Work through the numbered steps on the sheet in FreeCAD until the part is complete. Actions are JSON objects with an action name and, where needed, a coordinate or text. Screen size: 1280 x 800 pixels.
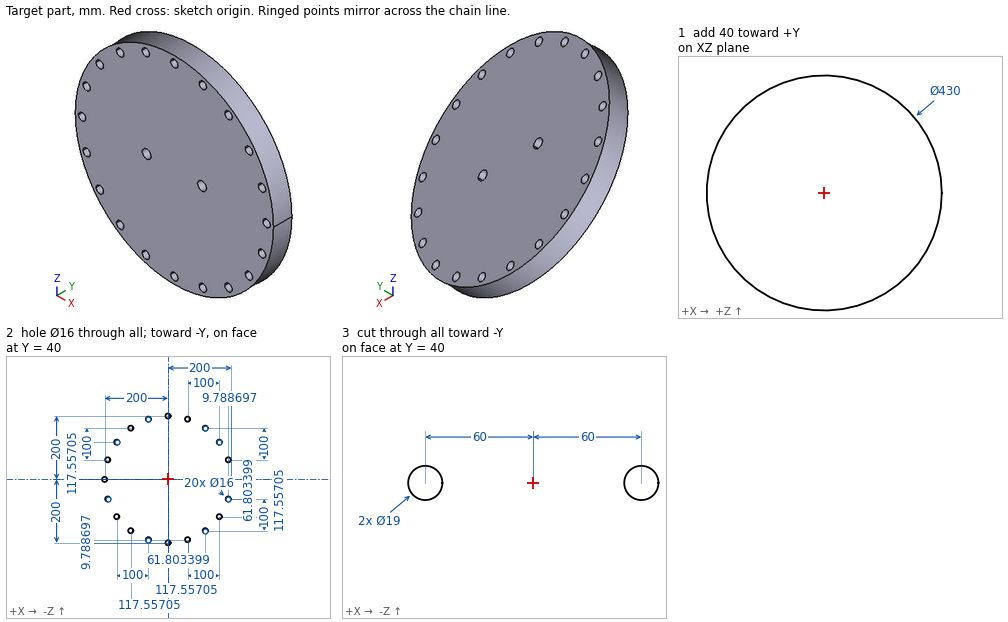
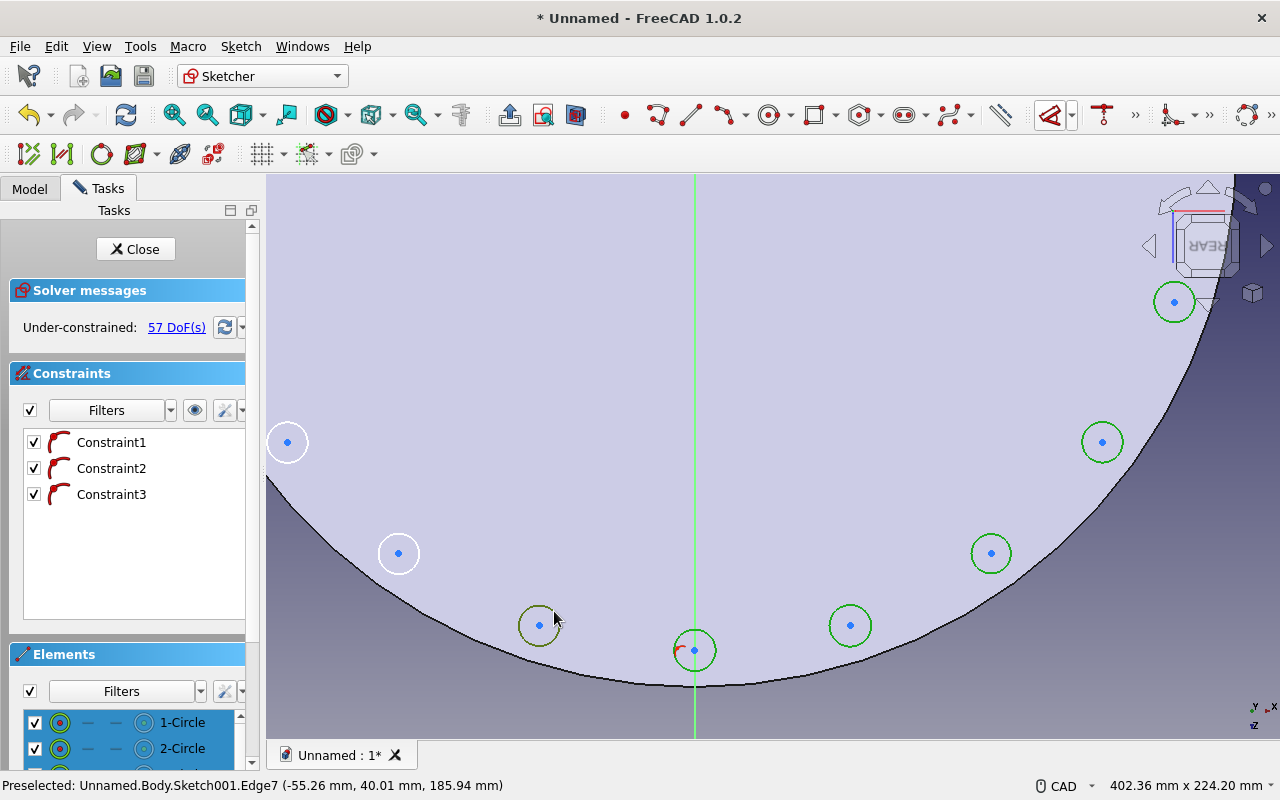
{"action": "left_click", "coordinate": [413, 540]}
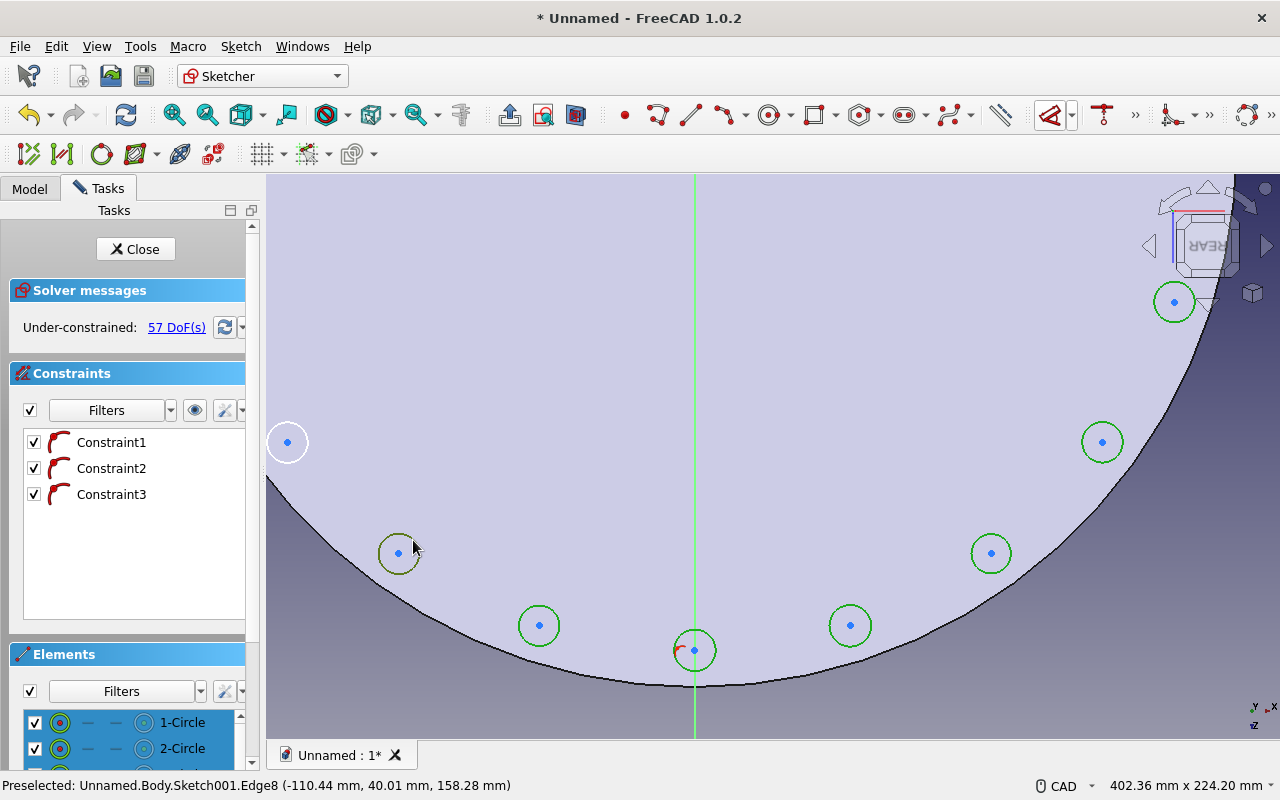
{"action": "left_click", "coordinate": [302, 428]}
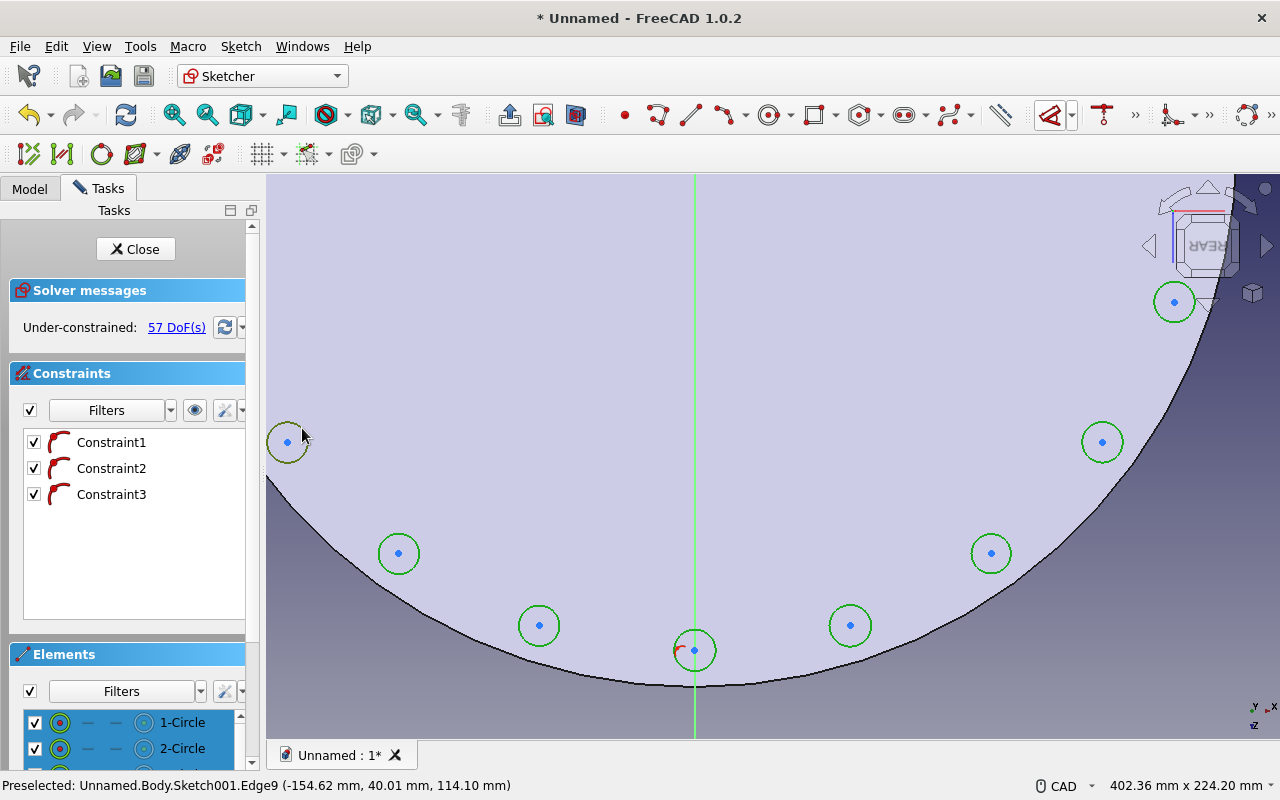
{"action": "scroll", "coordinate": [710, 638], "scroll_direction": "down", "scroll_amount": 5}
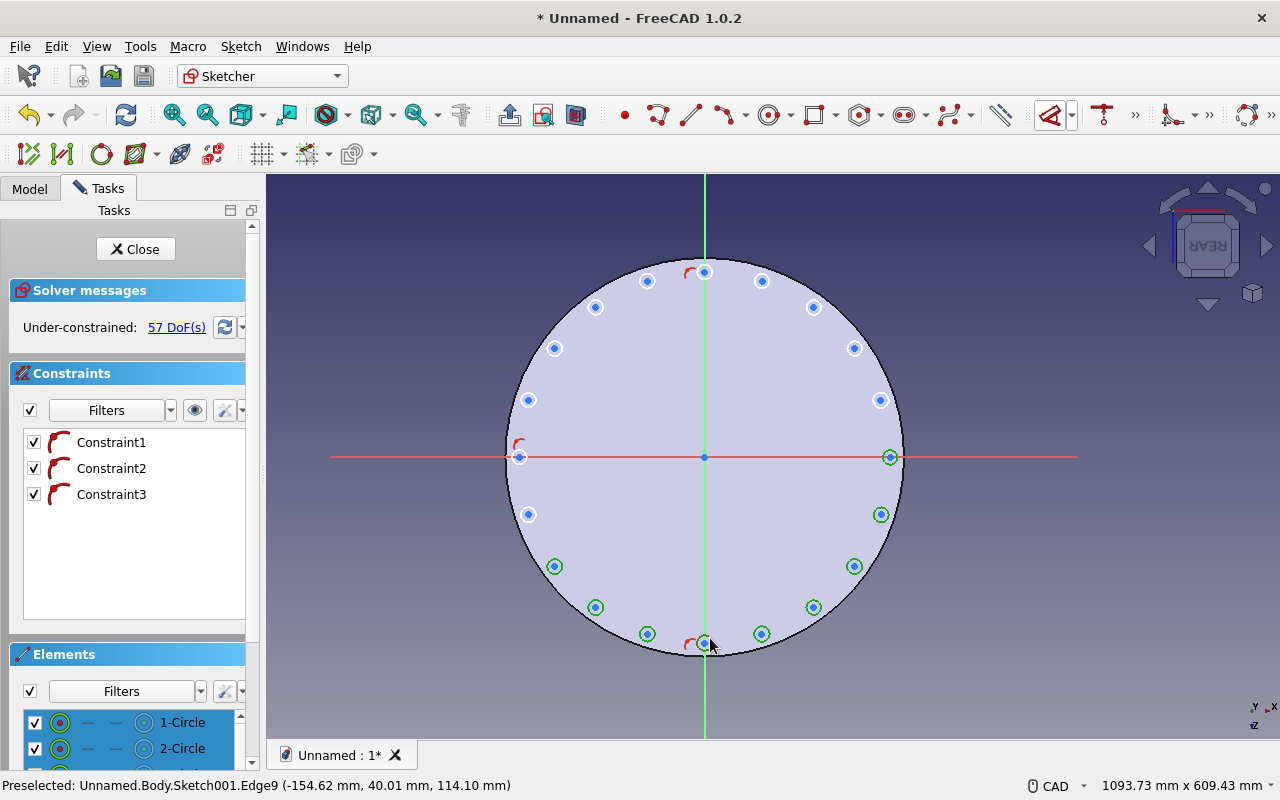
{"action": "scroll", "coordinate": [534, 510], "scroll_direction": "up", "scroll_amount": 4}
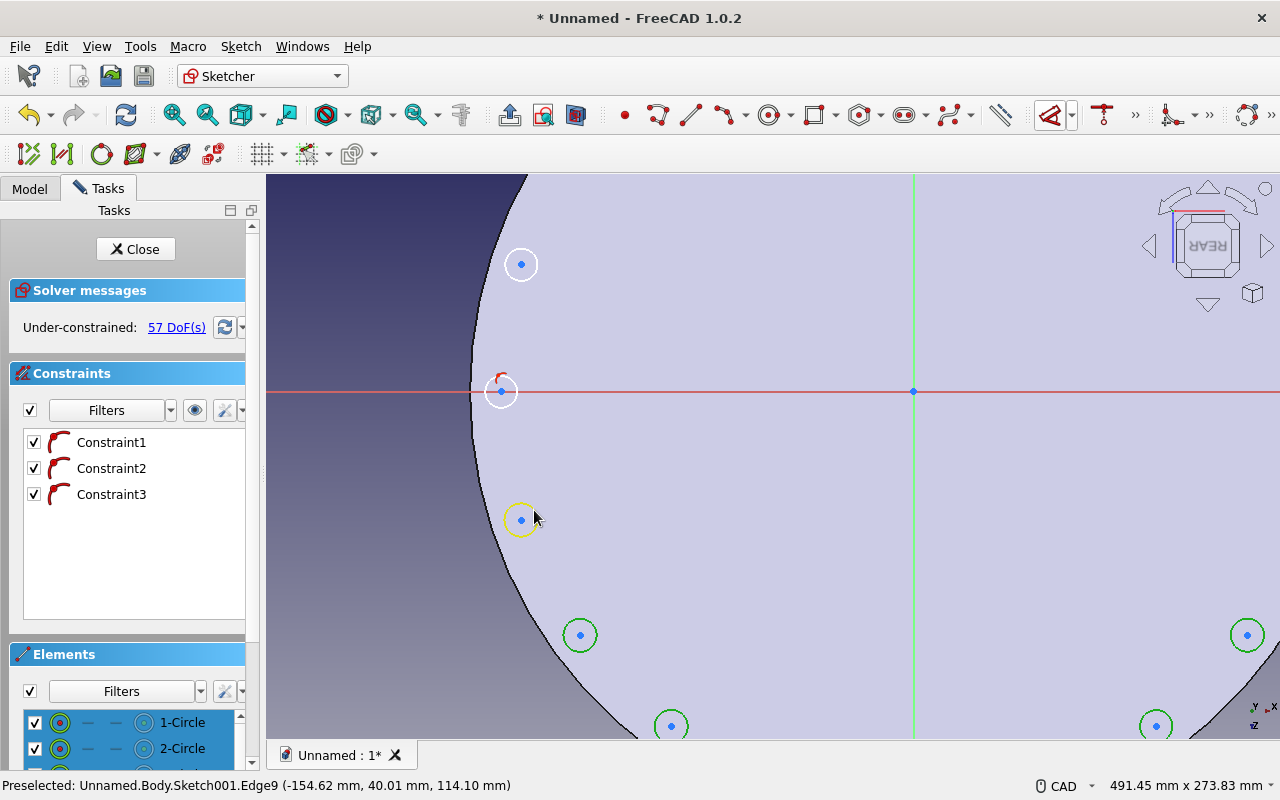
{"action": "left_click", "coordinate": [533, 508]}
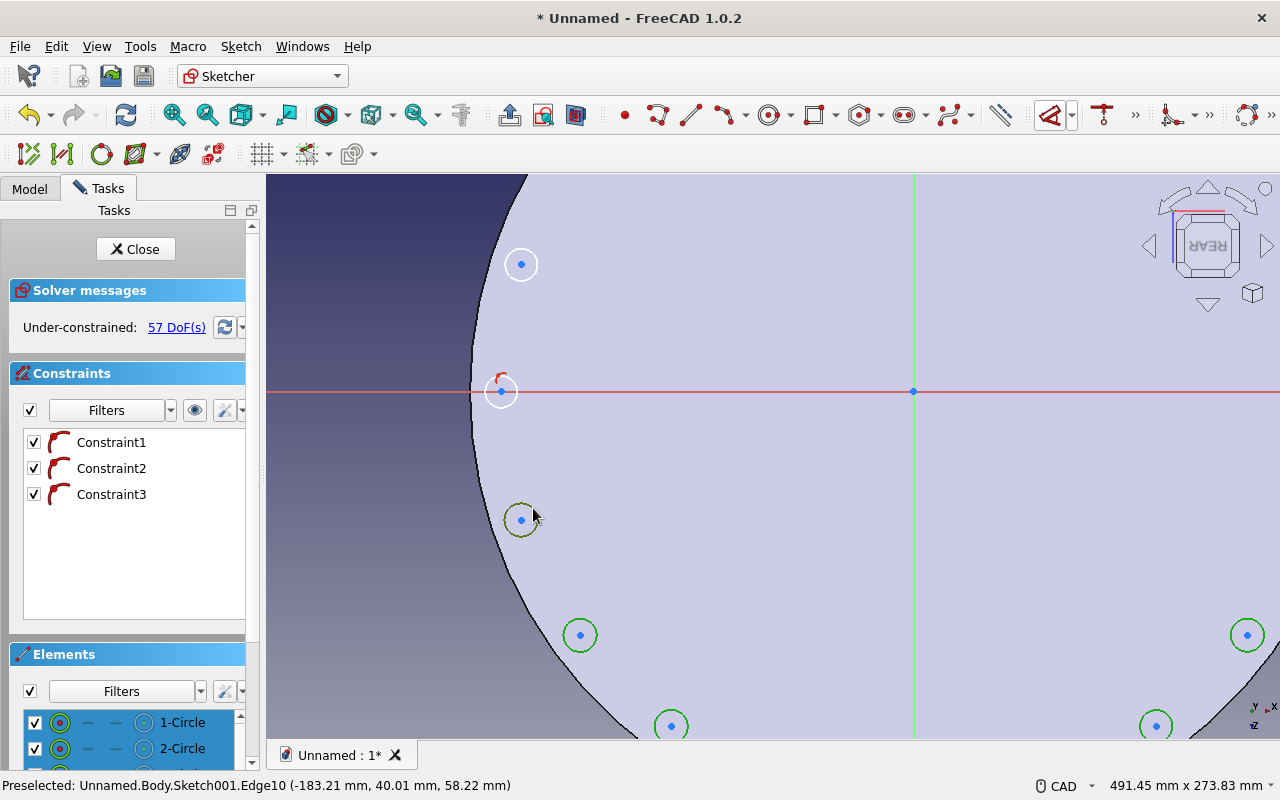
{"action": "scroll", "coordinate": [512, 381], "scroll_direction": "up", "scroll_amount": 2}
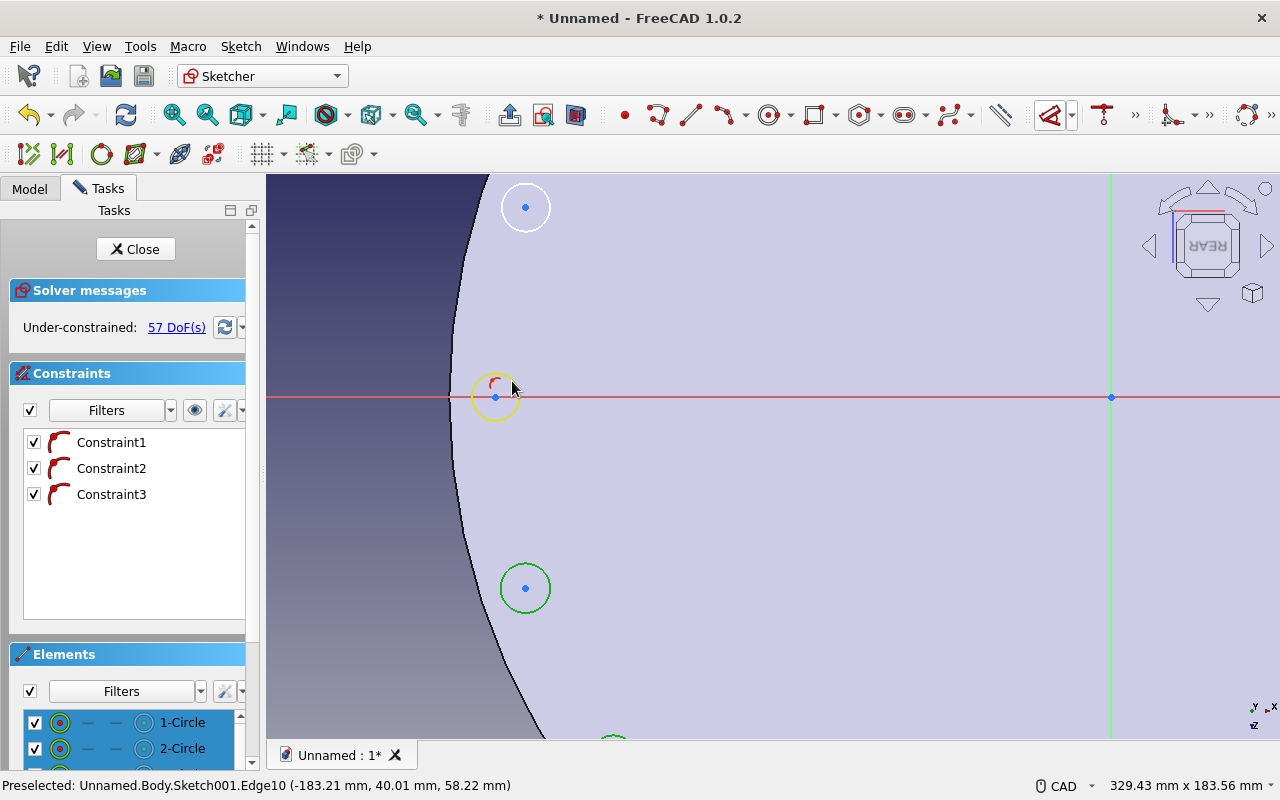
{"action": "left_click", "coordinate": [513, 380]}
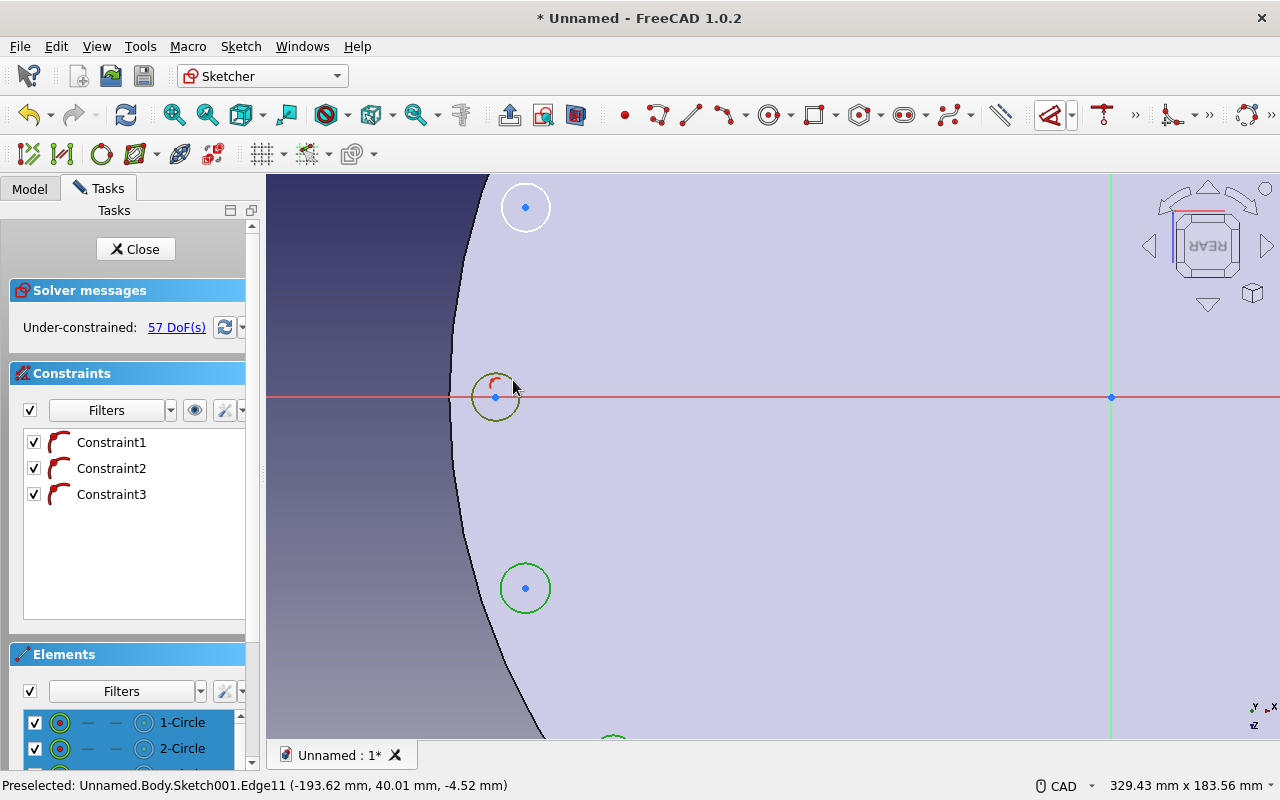
{"action": "left_click", "coordinate": [509, 225]}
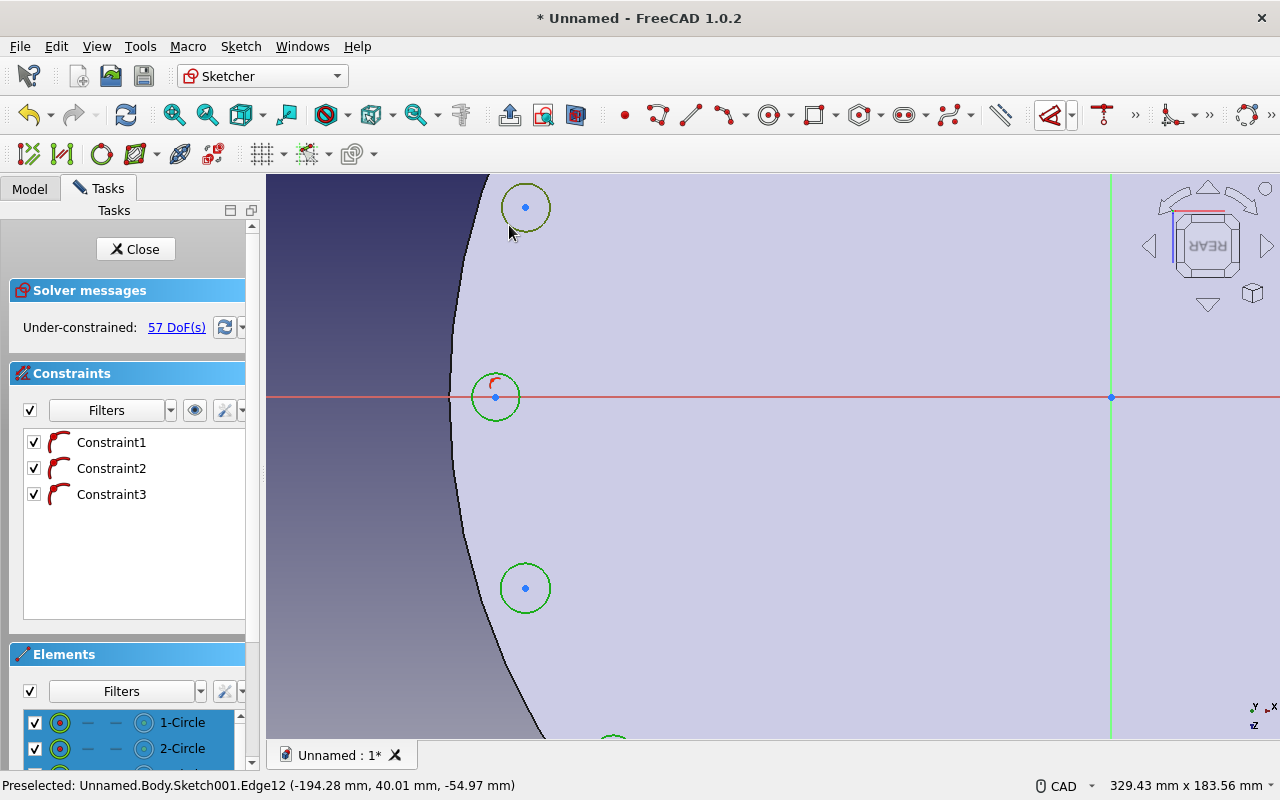
{"action": "scroll", "coordinate": [529, 482], "scroll_direction": "down", "scroll_amount": 6}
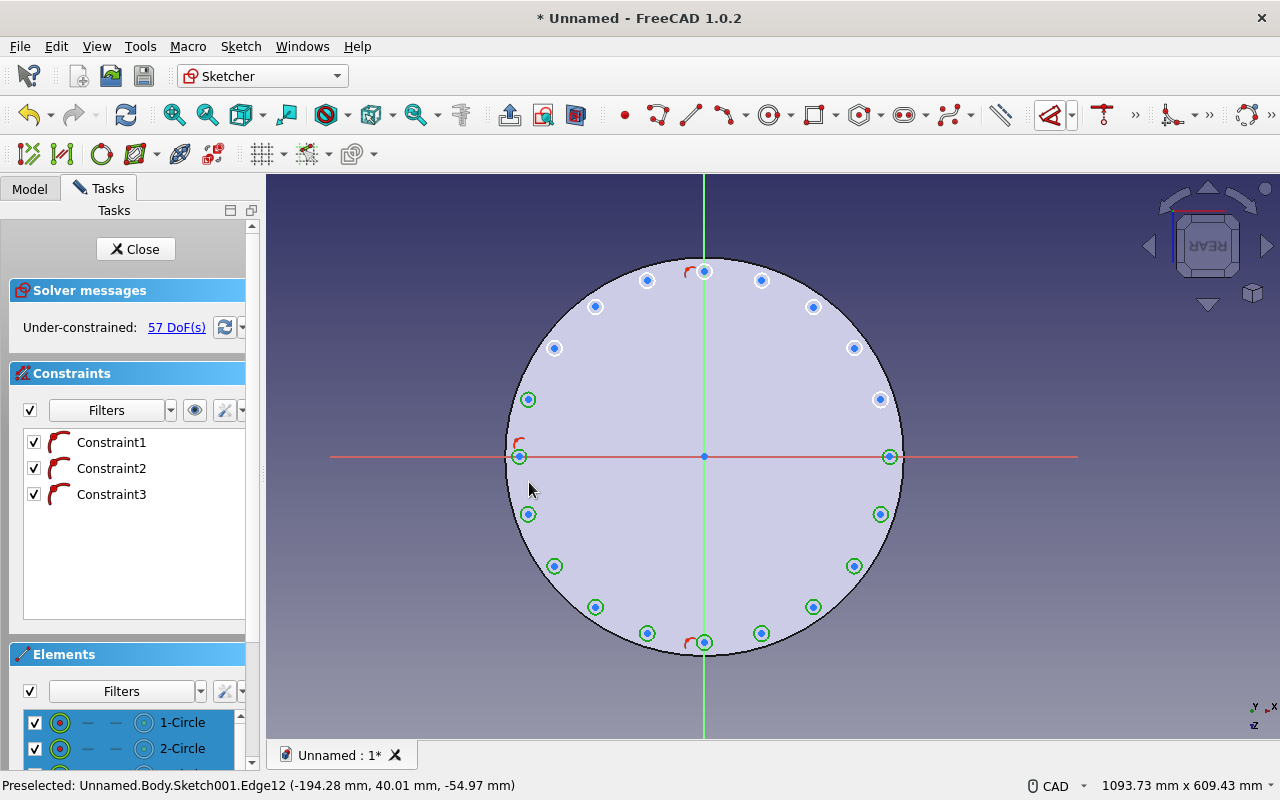
{"action": "scroll", "coordinate": [560, 343], "scroll_direction": "up", "scroll_amount": 4}